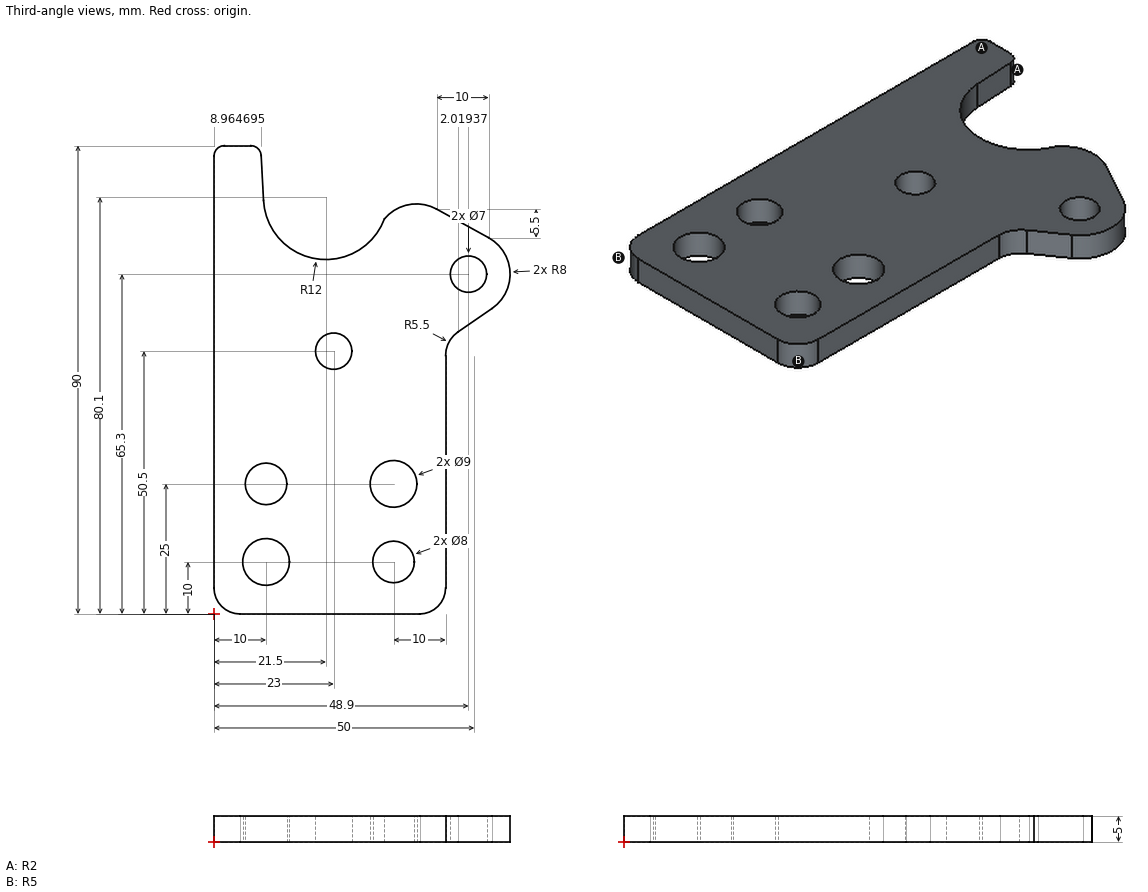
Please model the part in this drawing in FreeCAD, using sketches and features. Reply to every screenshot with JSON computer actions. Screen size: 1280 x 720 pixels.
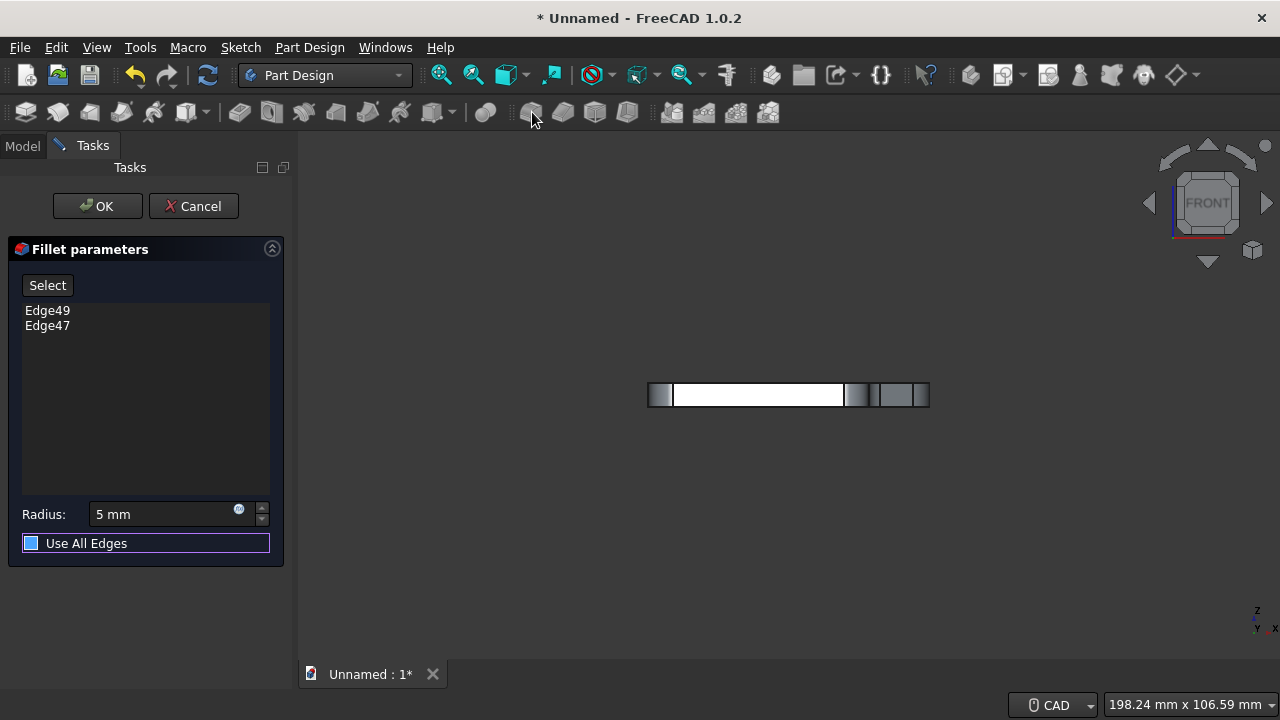
{"action": "left_click", "coordinate": [98, 206]}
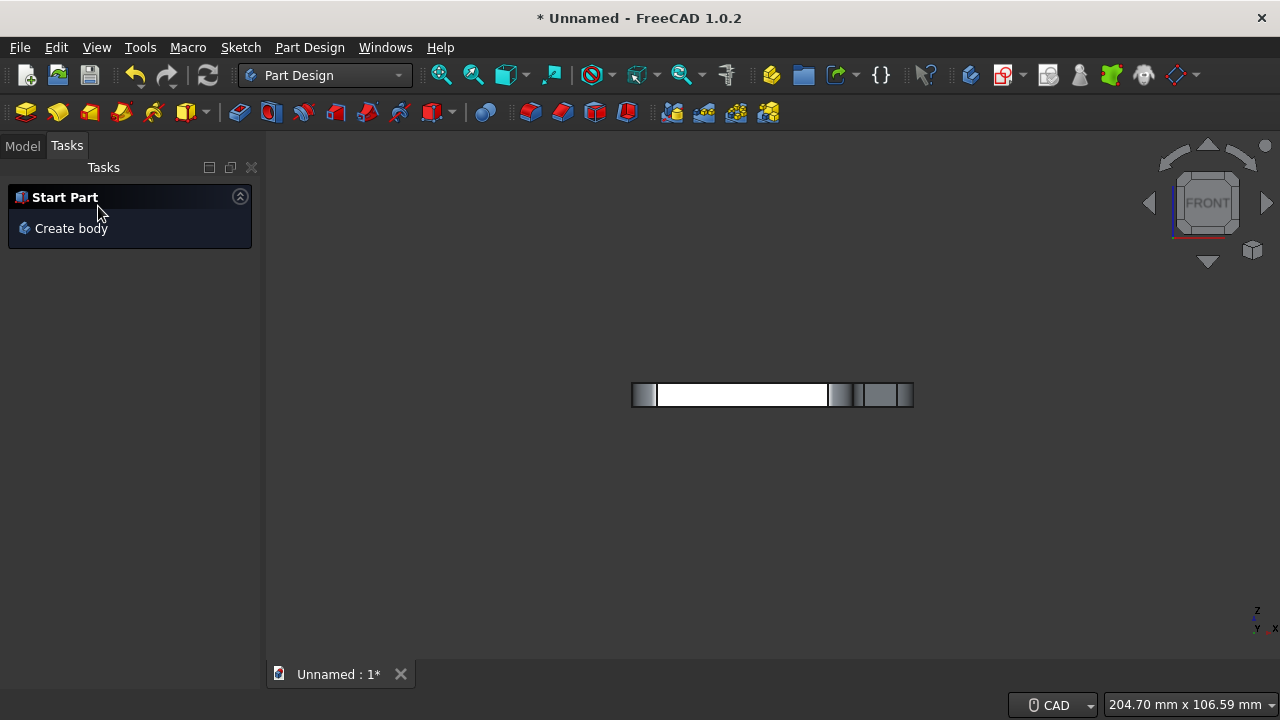
{"action": "key", "text": "0"}